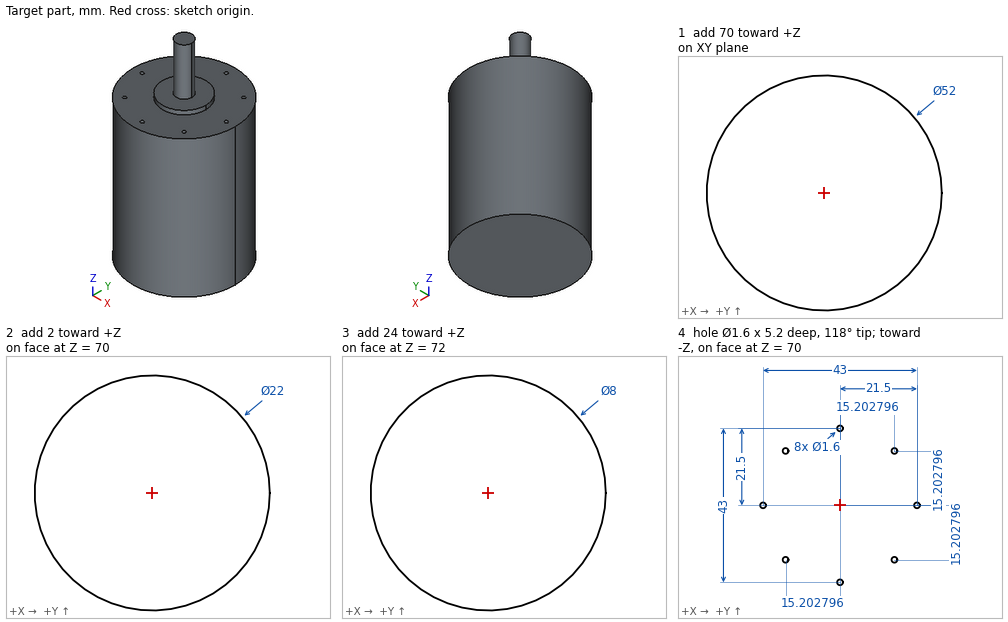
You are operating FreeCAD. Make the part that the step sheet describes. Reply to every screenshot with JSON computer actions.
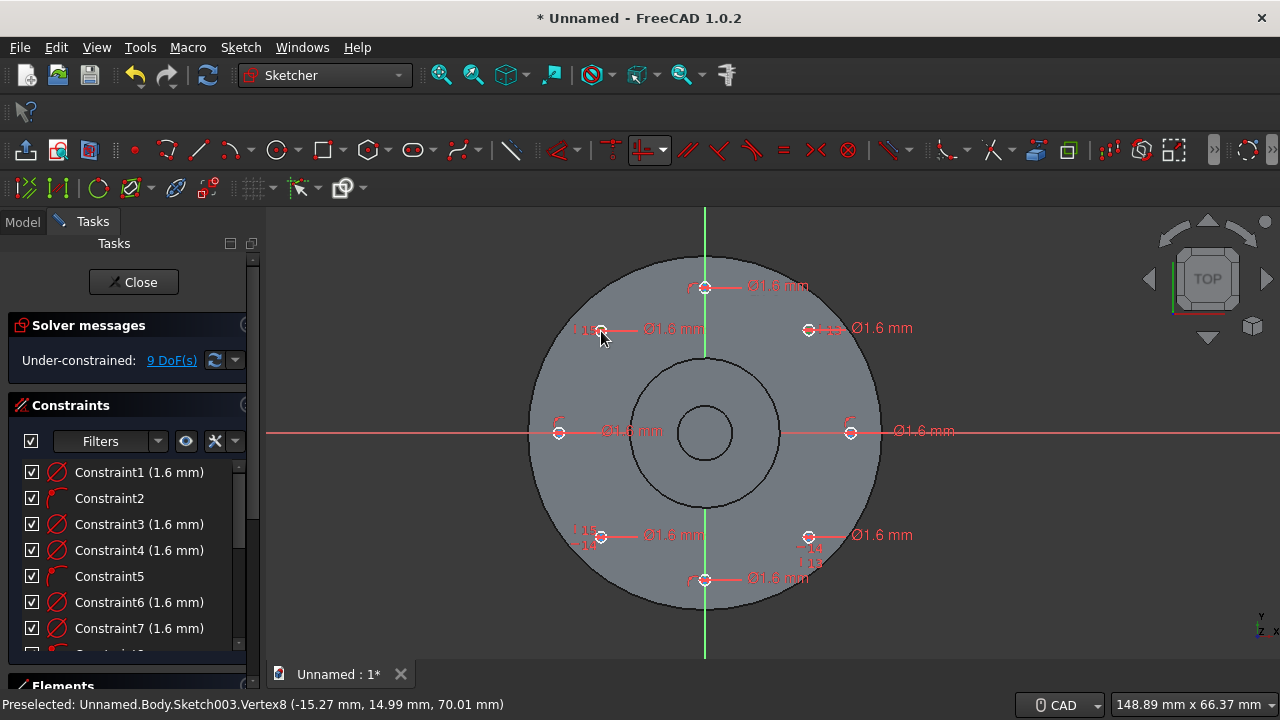
{"action": "key", "text": "h"}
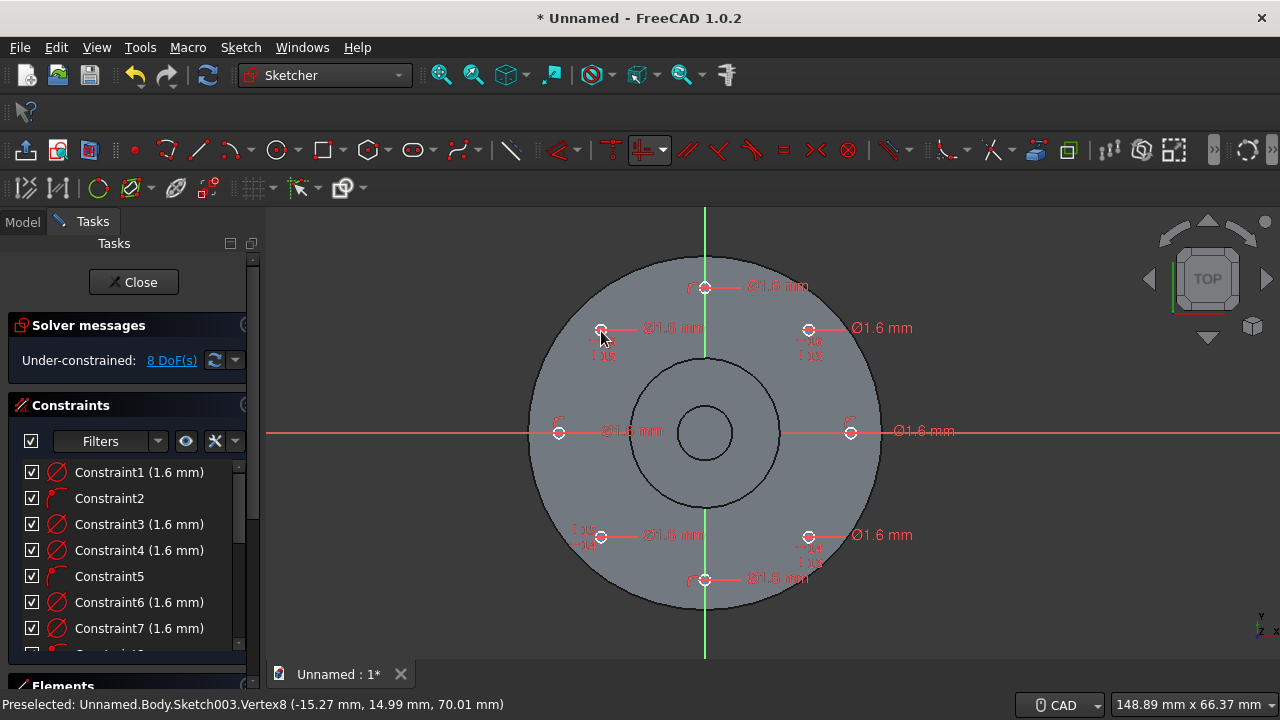
{"action": "left_click", "coordinate": [558, 150]}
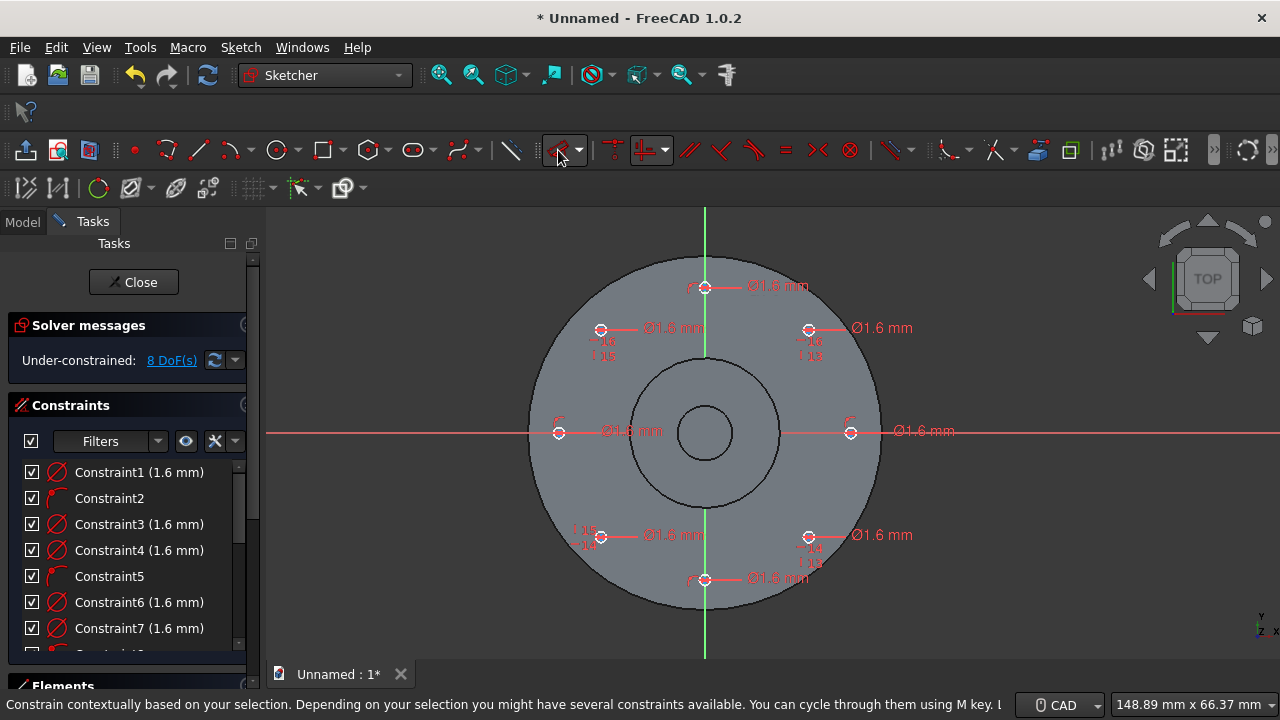
{"action": "left_click", "coordinate": [705, 288]}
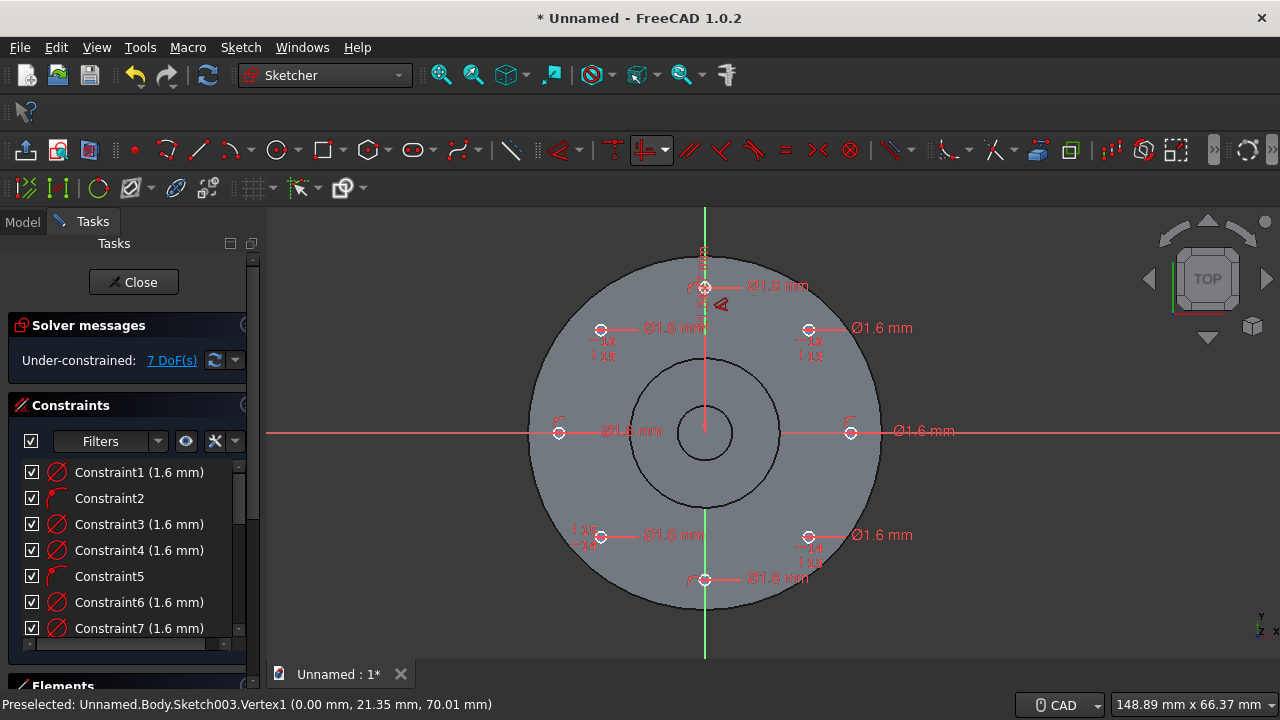
{"action": "left_click", "coordinate": [705, 580]}
{"action": "left_click", "coordinate": [739, 367]}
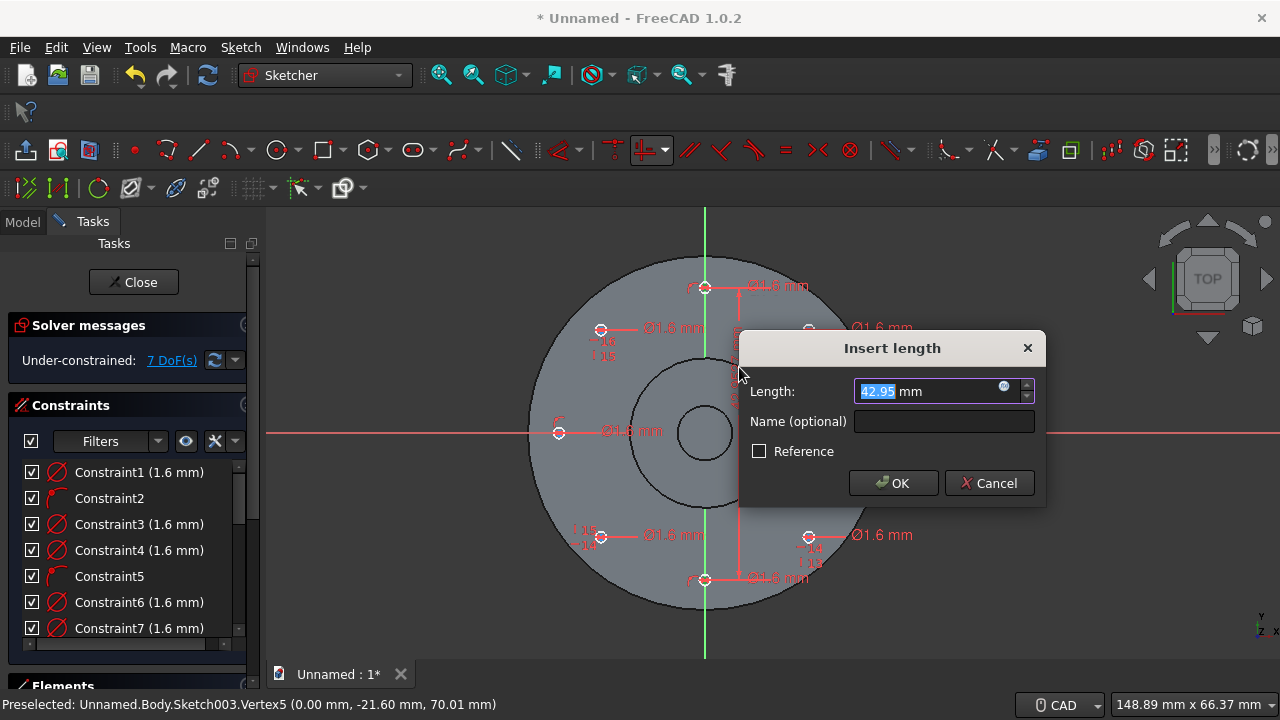
{"action": "type", "text": "43"}
{"action": "key", "text": "Return"}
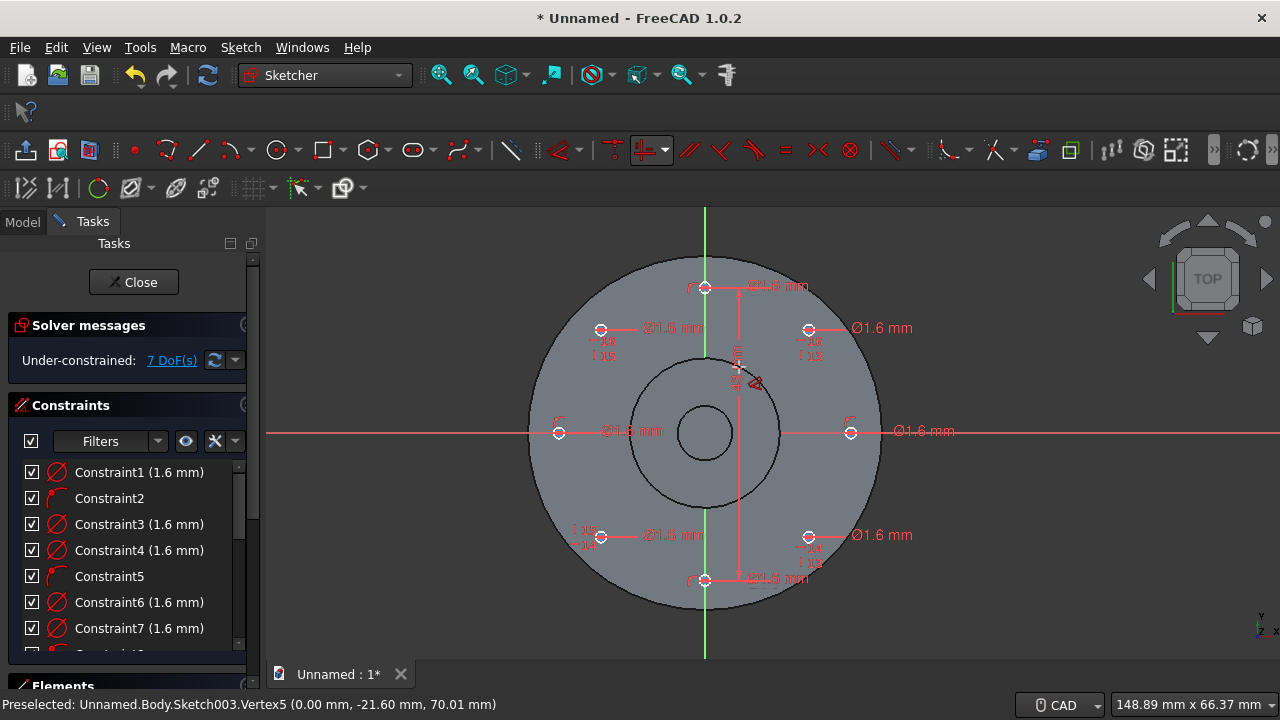
{"action": "left_click", "coordinate": [851, 433]}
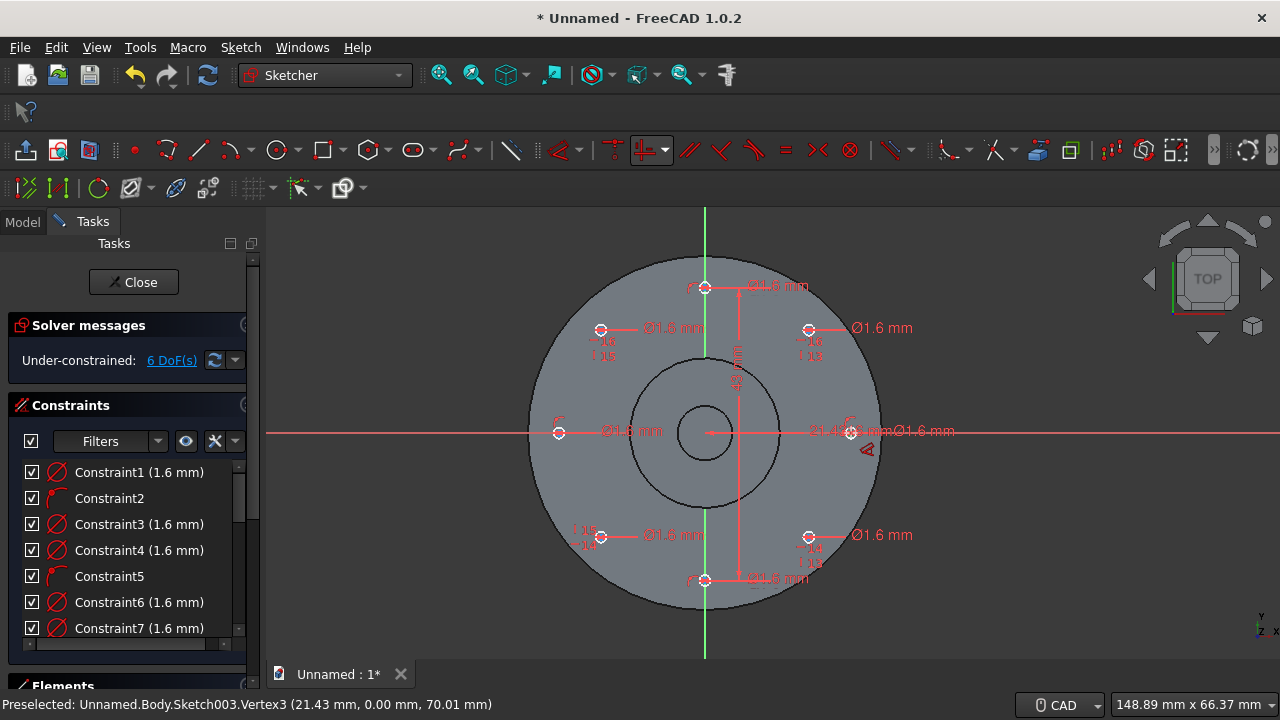
{"action": "left_click", "coordinate": [559, 433]}
{"action": "left_click", "coordinate": [638, 467]}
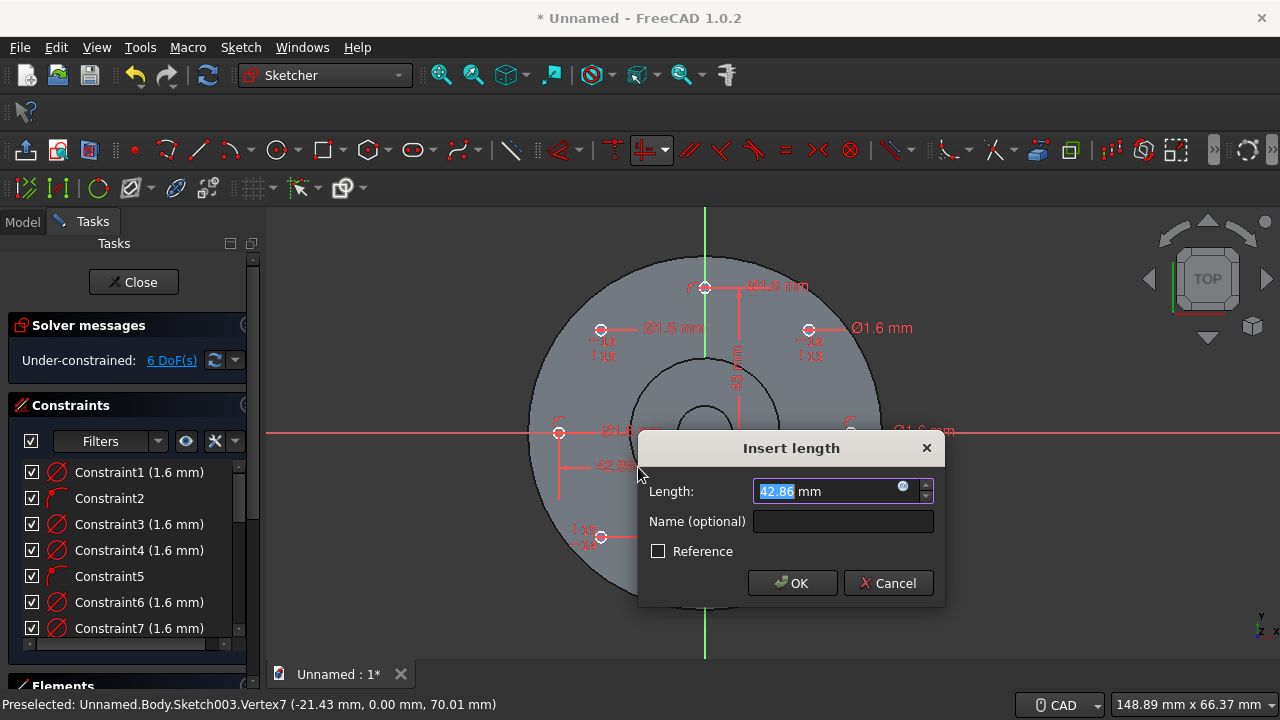
{"action": "type", "text": "43"}
{"action": "key", "text": "Return"}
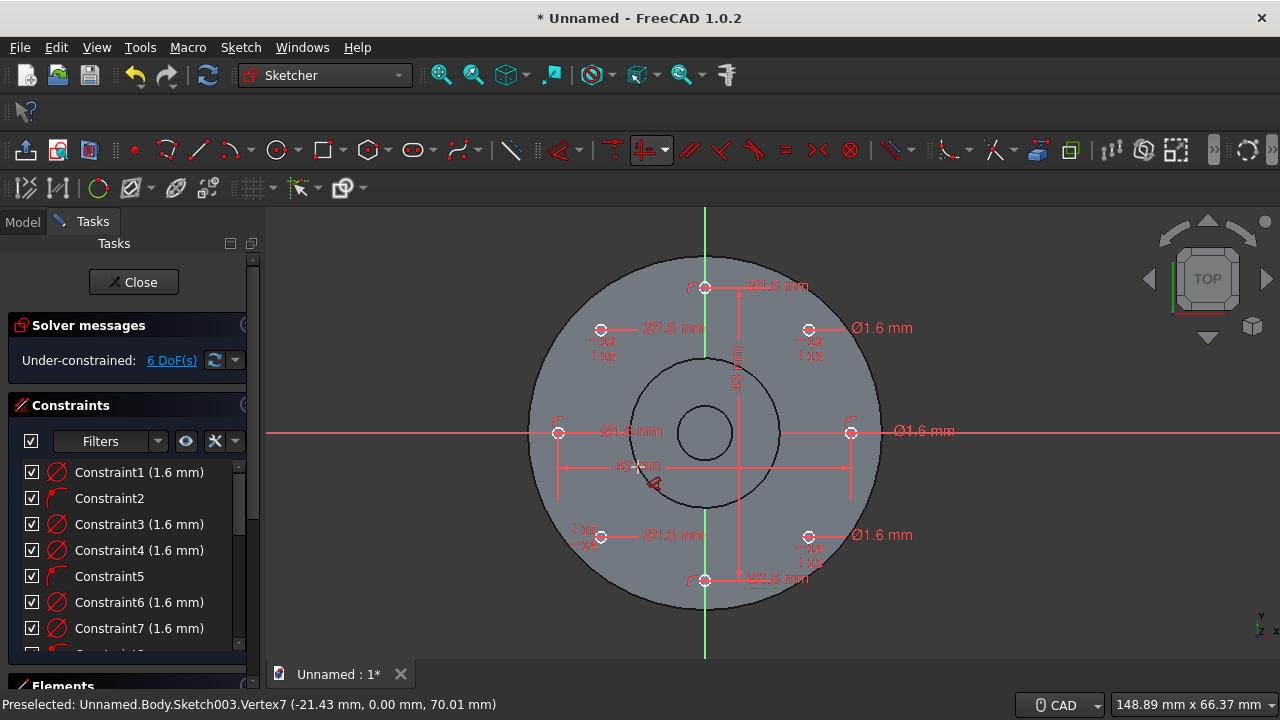
{"action": "left_click", "coordinate": [705, 288]}
{"action": "left_click", "coordinate": [739, 327]}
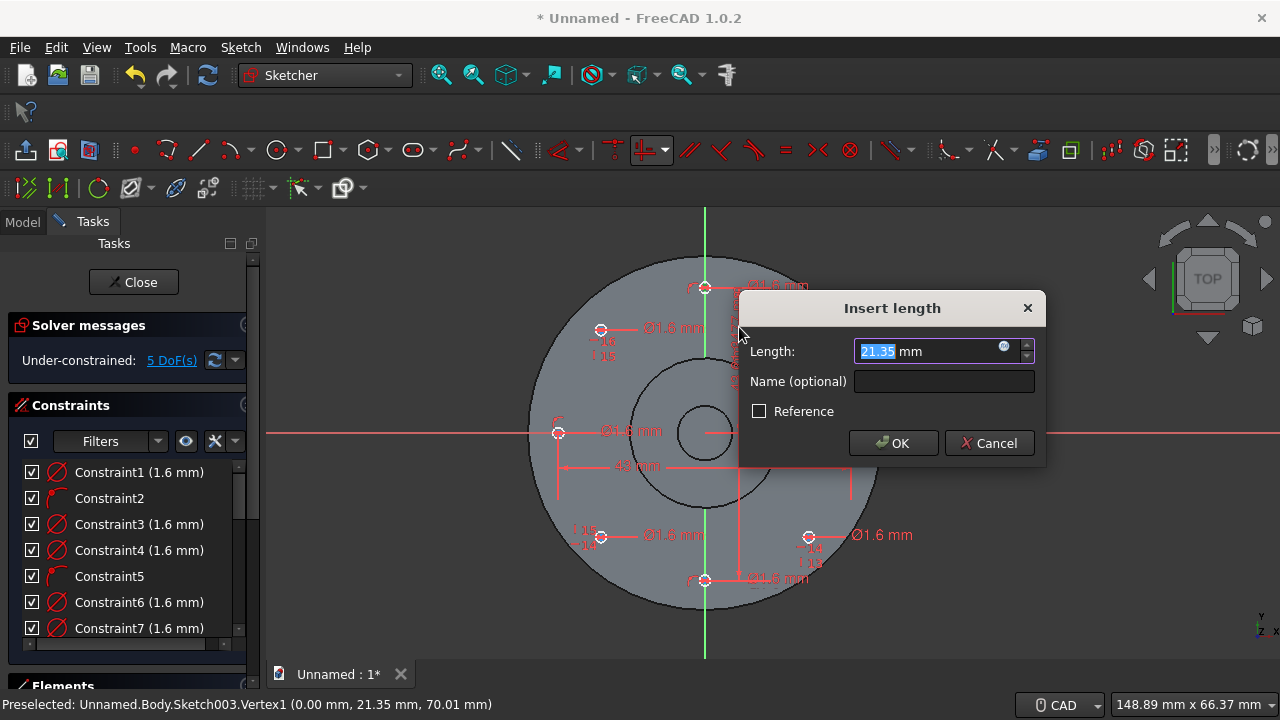
{"action": "type", "text": "21.5"}
{"action": "key", "text": "Return"}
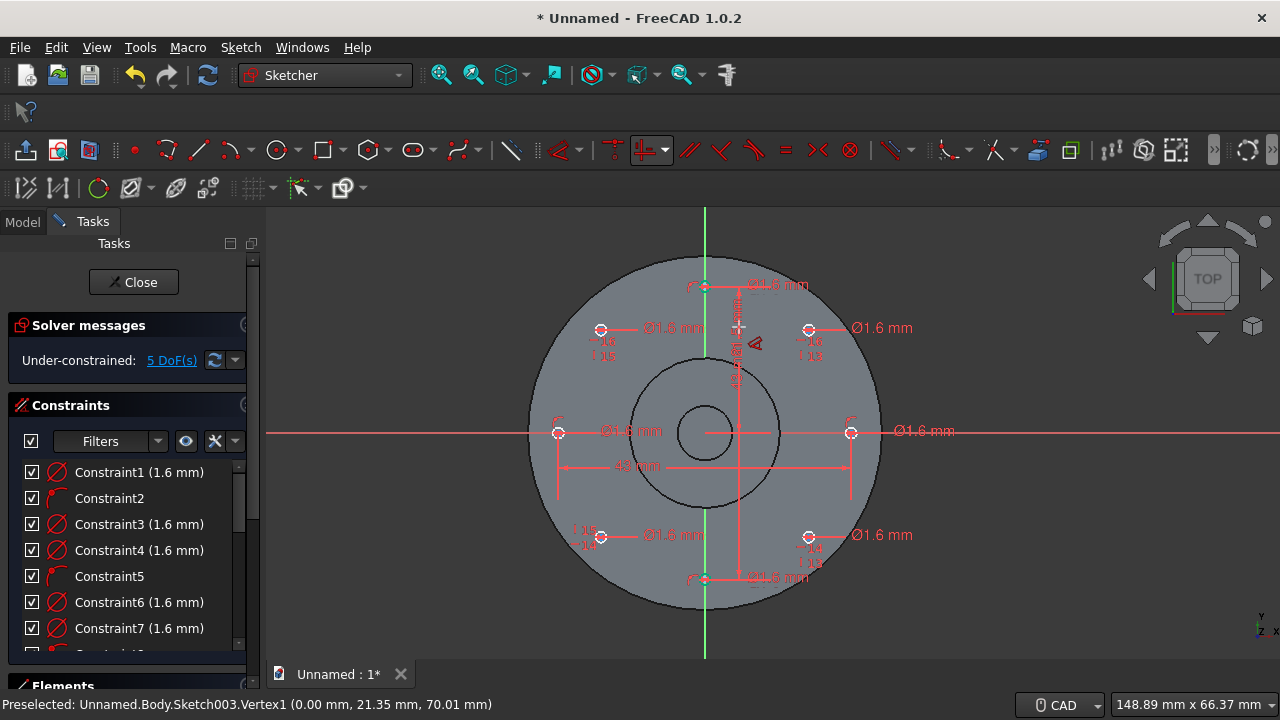
{"action": "left_click", "coordinate": [851, 433]}
{"action": "left_click", "coordinate": [778, 467]}